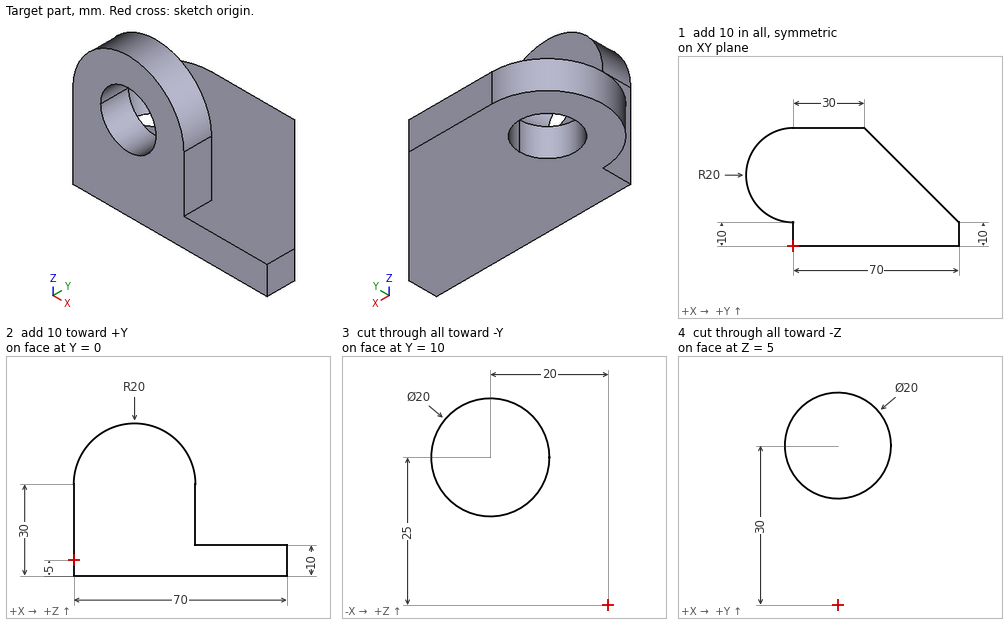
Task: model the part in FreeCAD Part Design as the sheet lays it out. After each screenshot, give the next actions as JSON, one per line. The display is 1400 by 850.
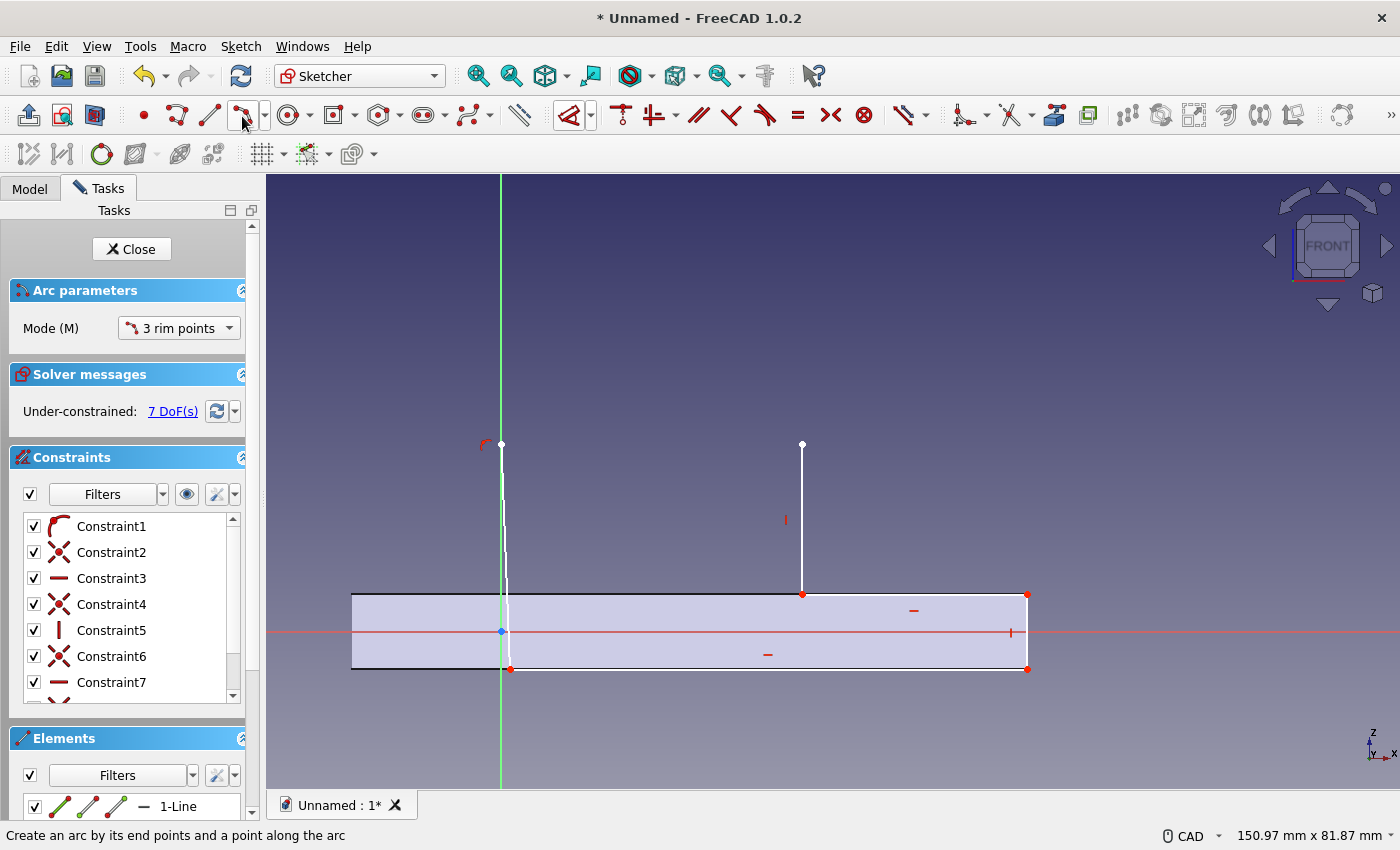
{"action": "left_click", "coordinate": [802, 445]}
{"action": "left_click", "coordinate": [501, 445]}
{"action": "left_click", "coordinate": [652, 294]}
{"action": "key", "text": "Escape"}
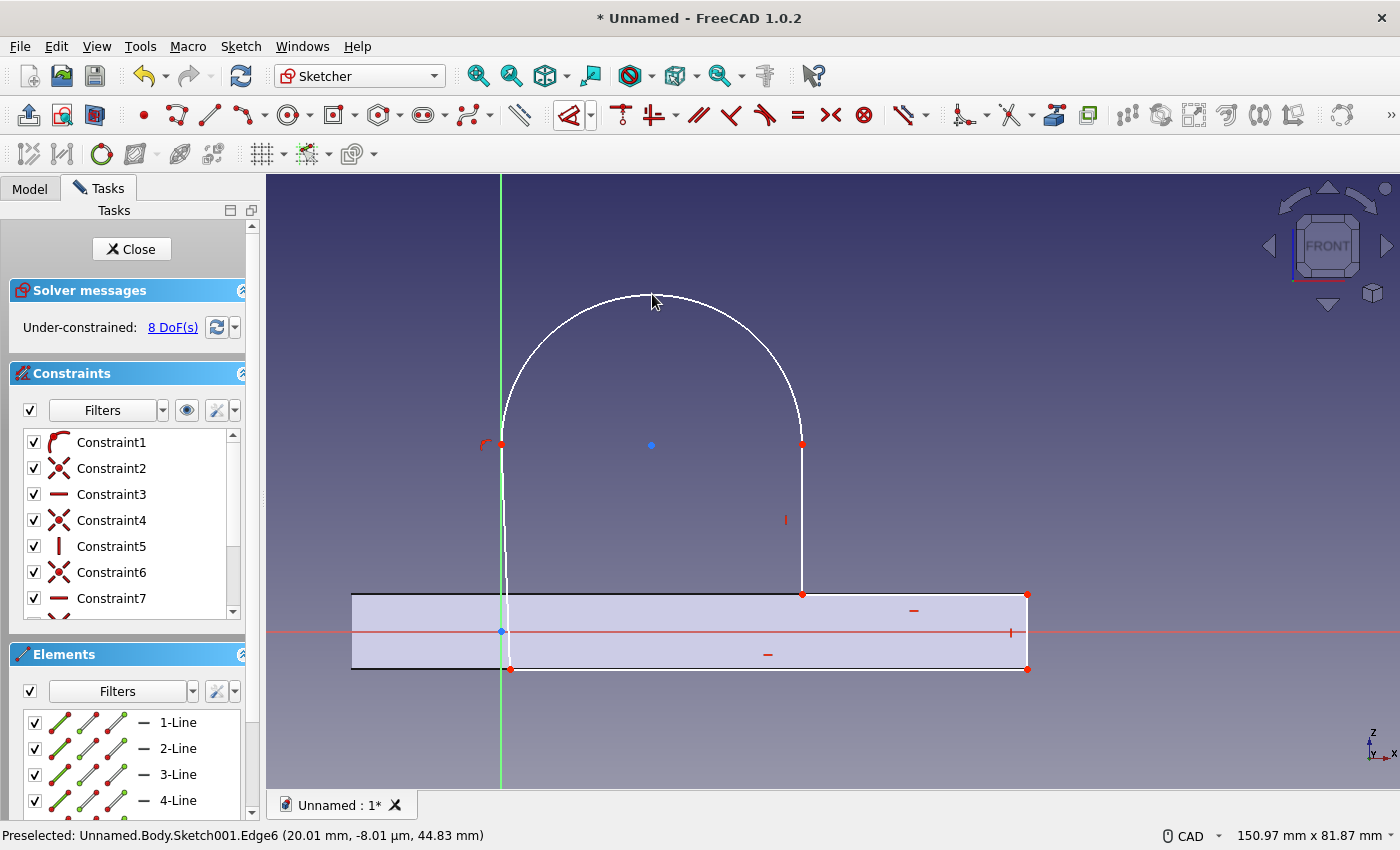
{"action": "left_click", "coordinate": [504, 512]}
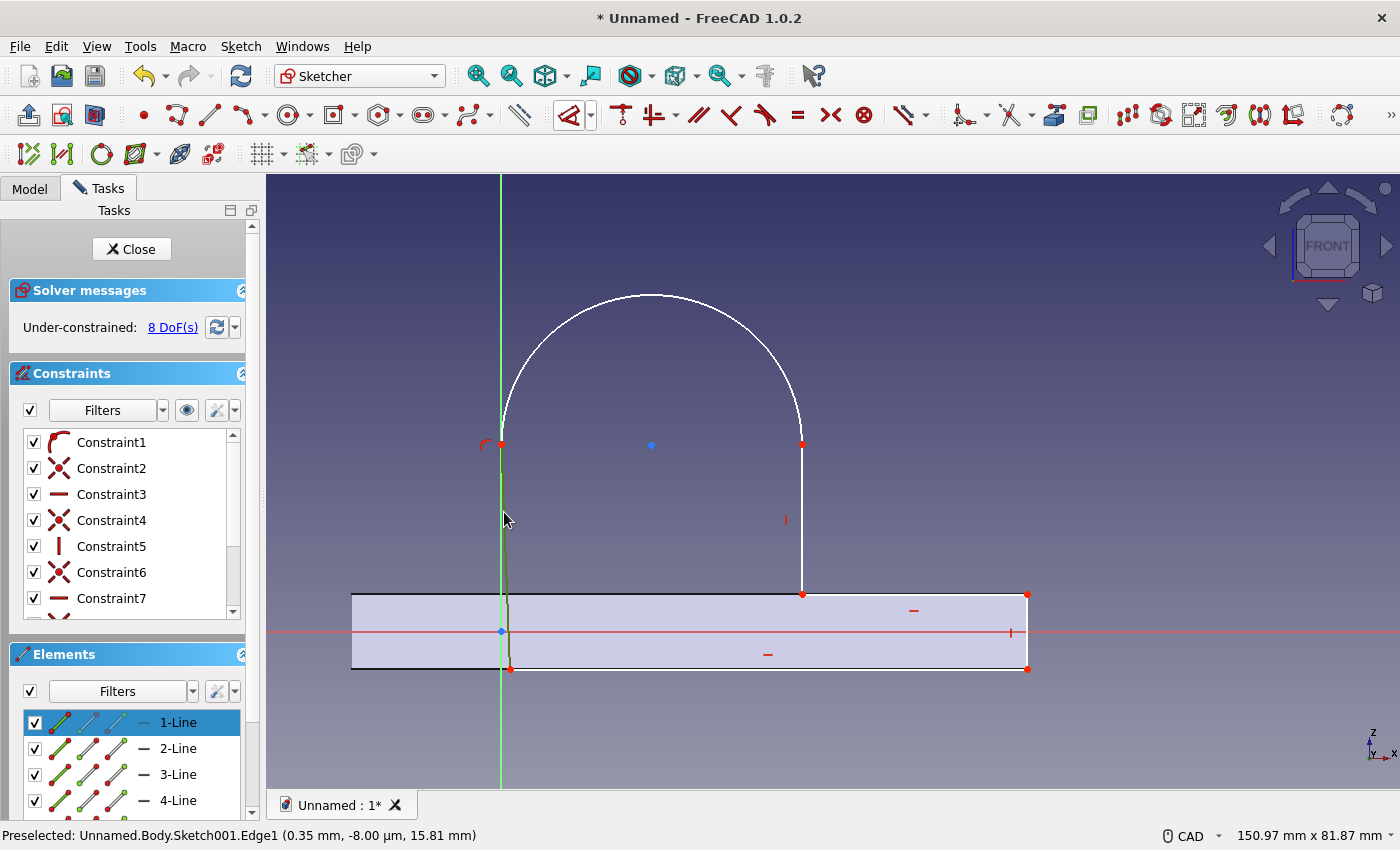
{"action": "left_click", "coordinate": [740, 324]}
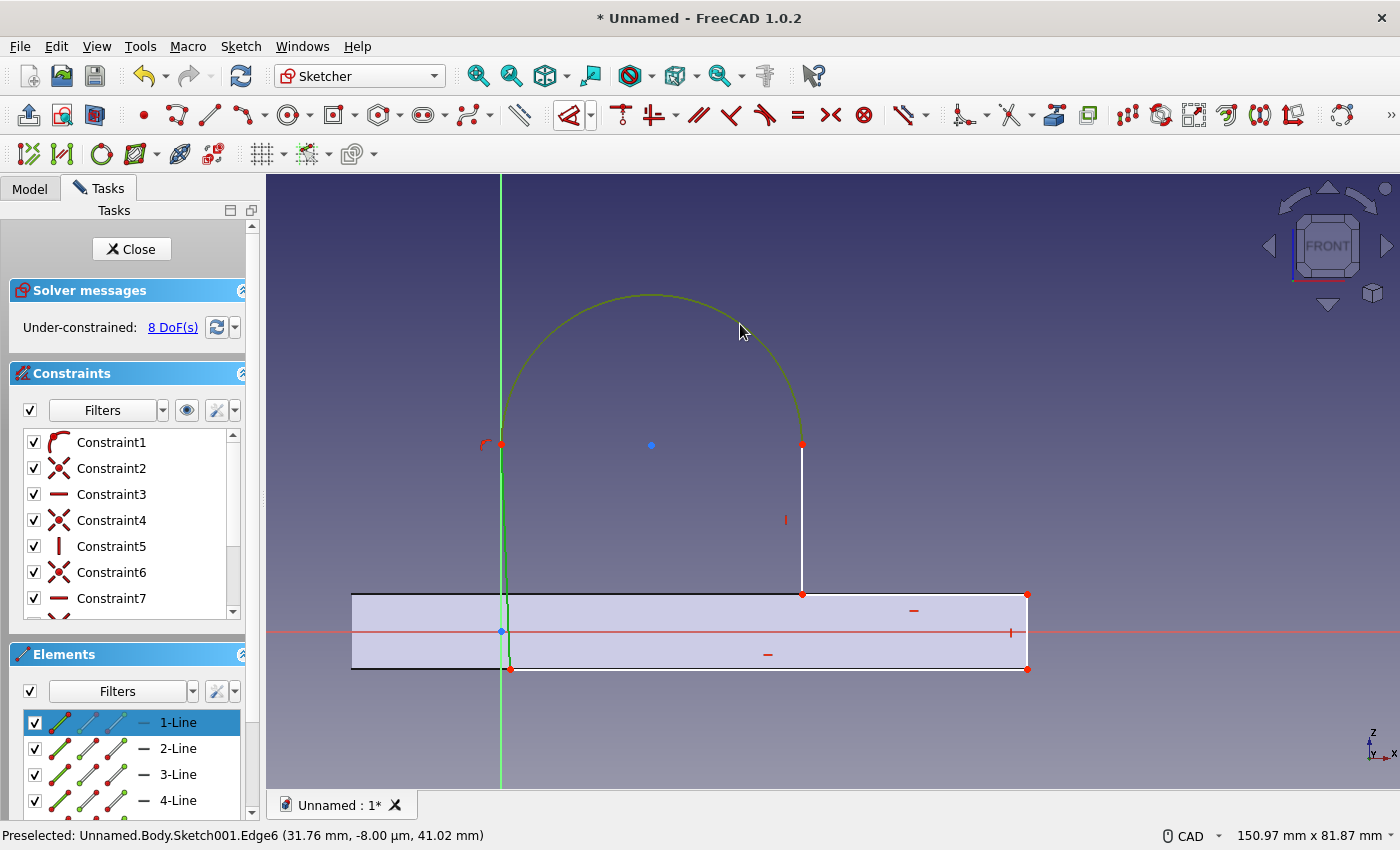
{"action": "left_click", "coordinate": [765, 116]}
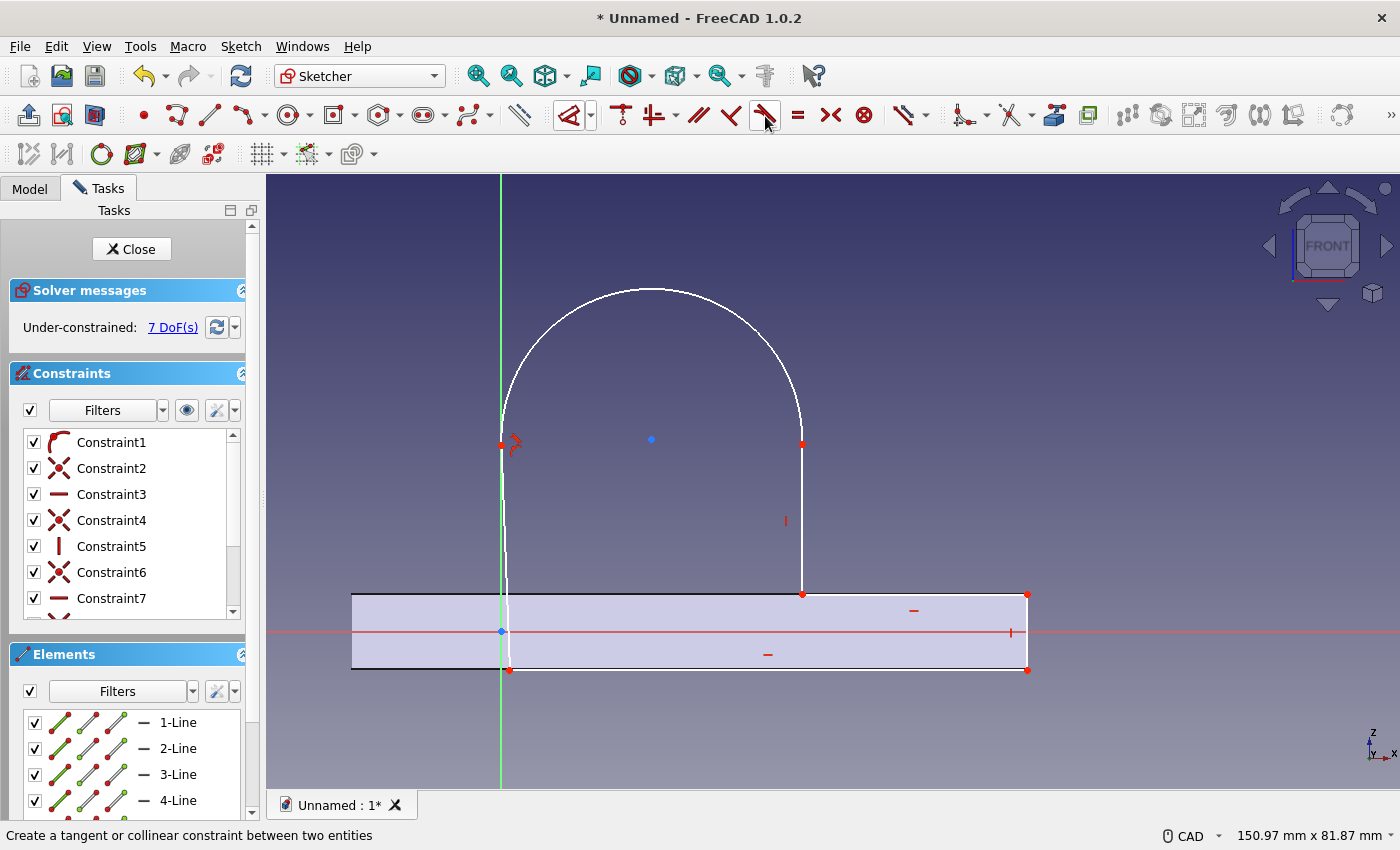
{"action": "left_click", "coordinate": [802, 550]}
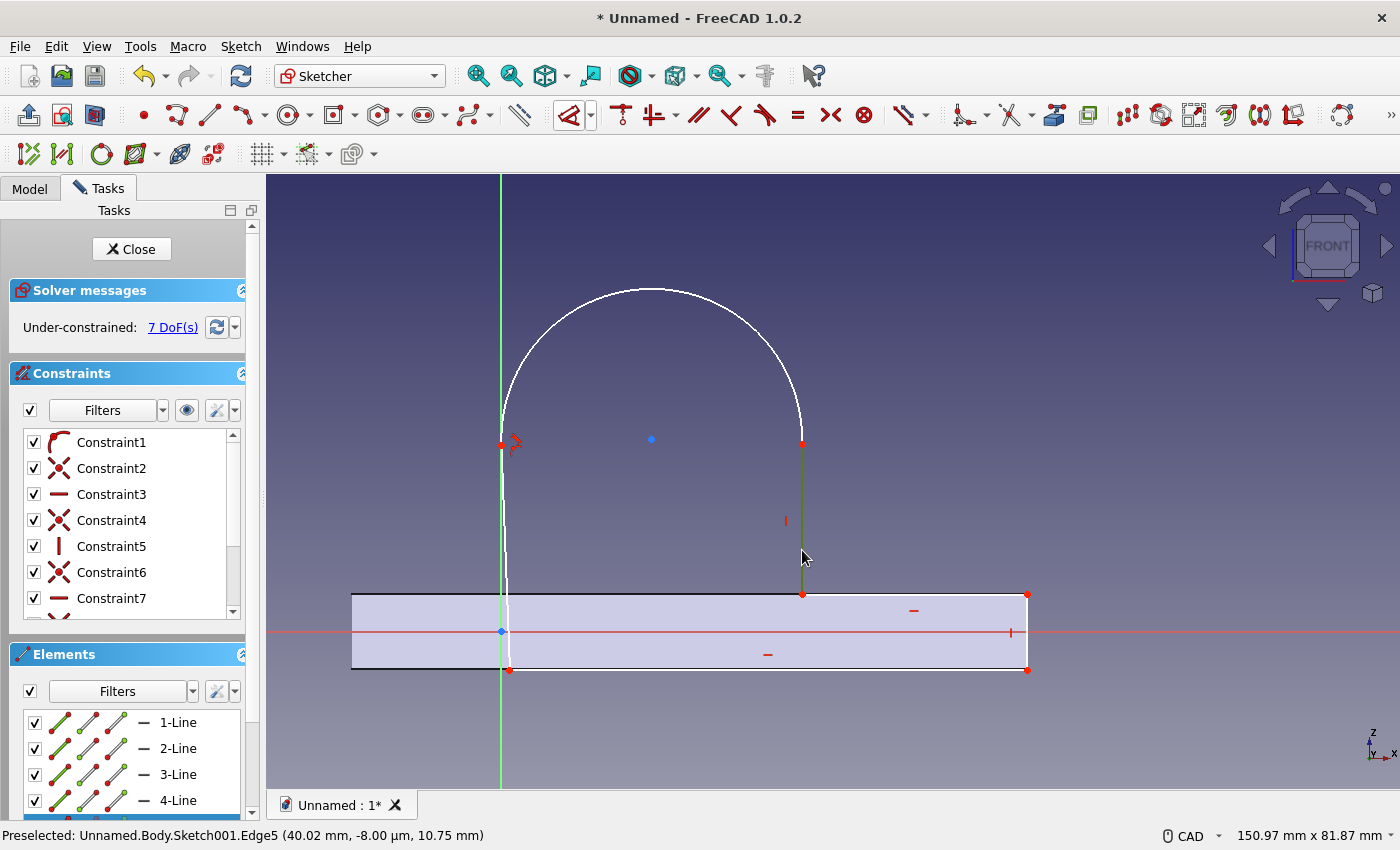
{"action": "left_click", "coordinate": [742, 319]}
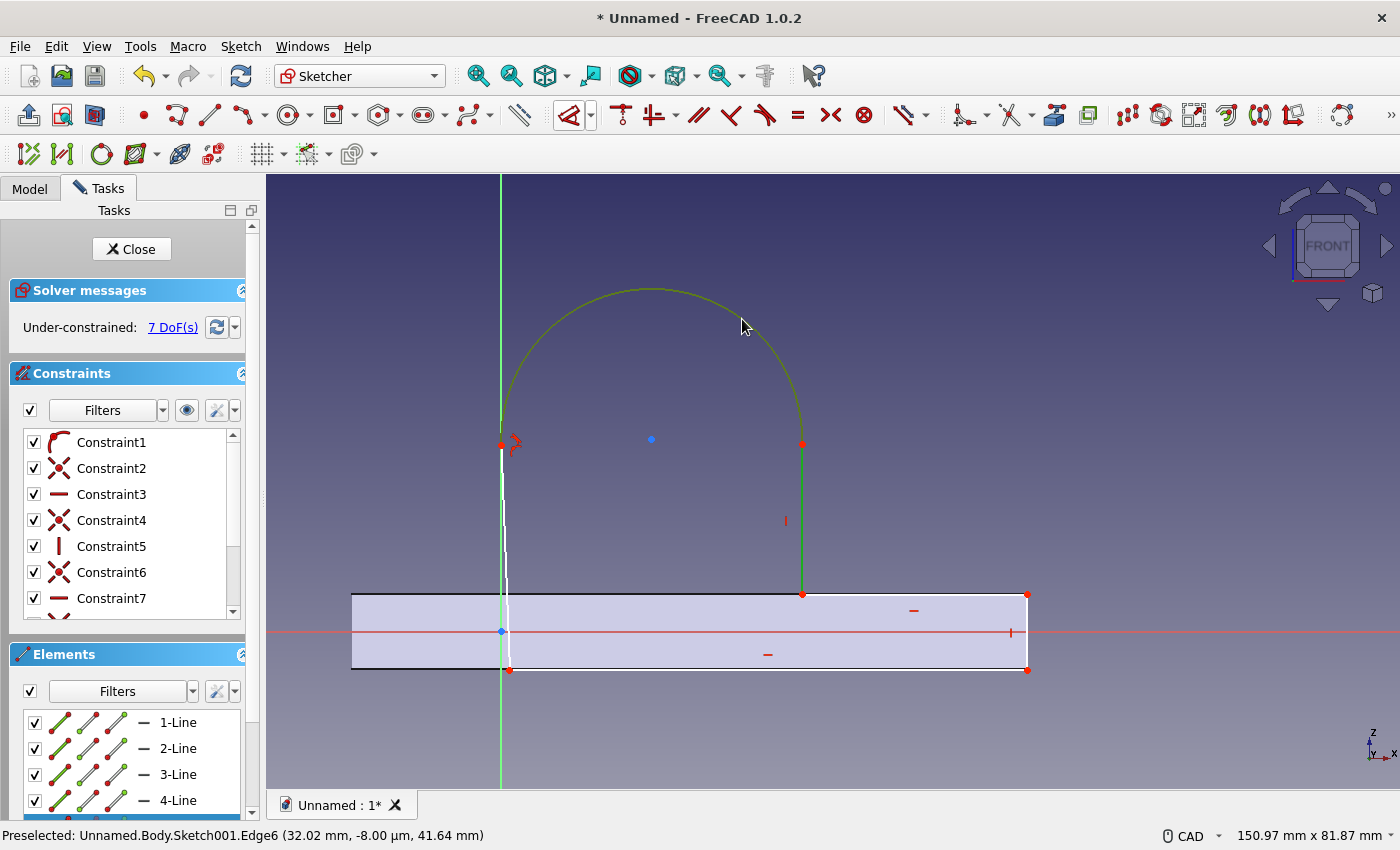
{"action": "left_click", "coordinate": [765, 116]}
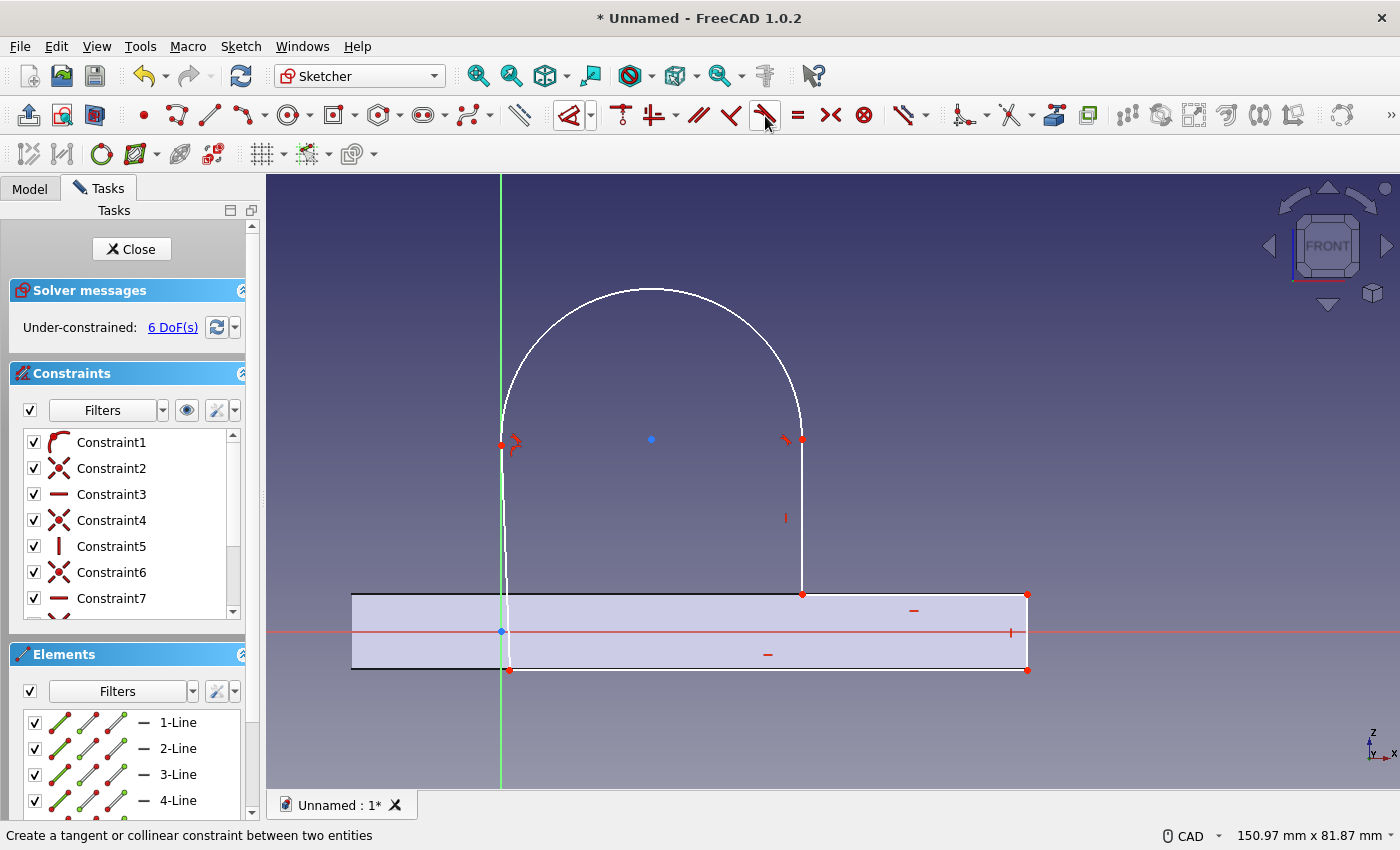
{"action": "left_click", "coordinate": [504, 513]}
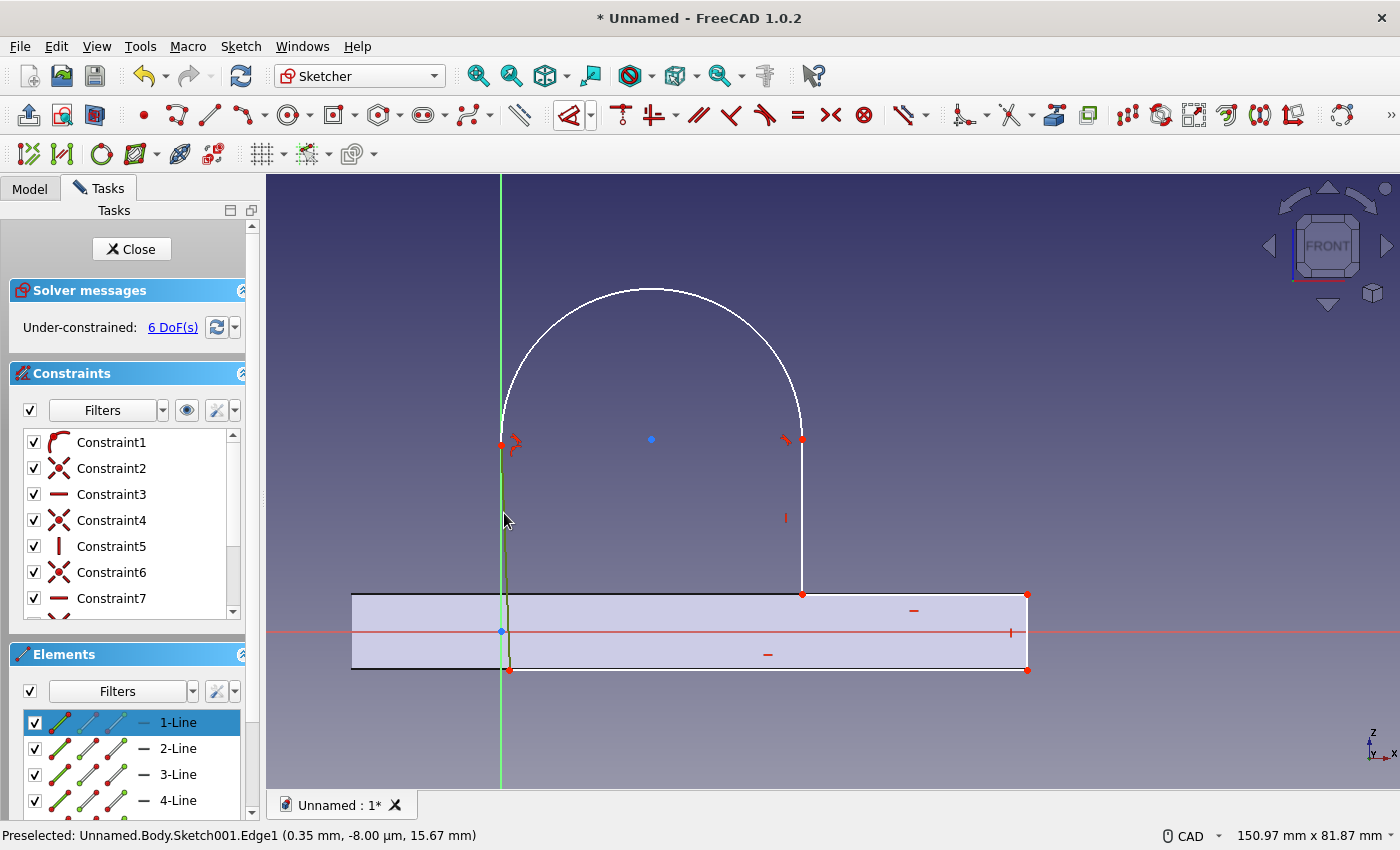
{"action": "key", "text": "v"}